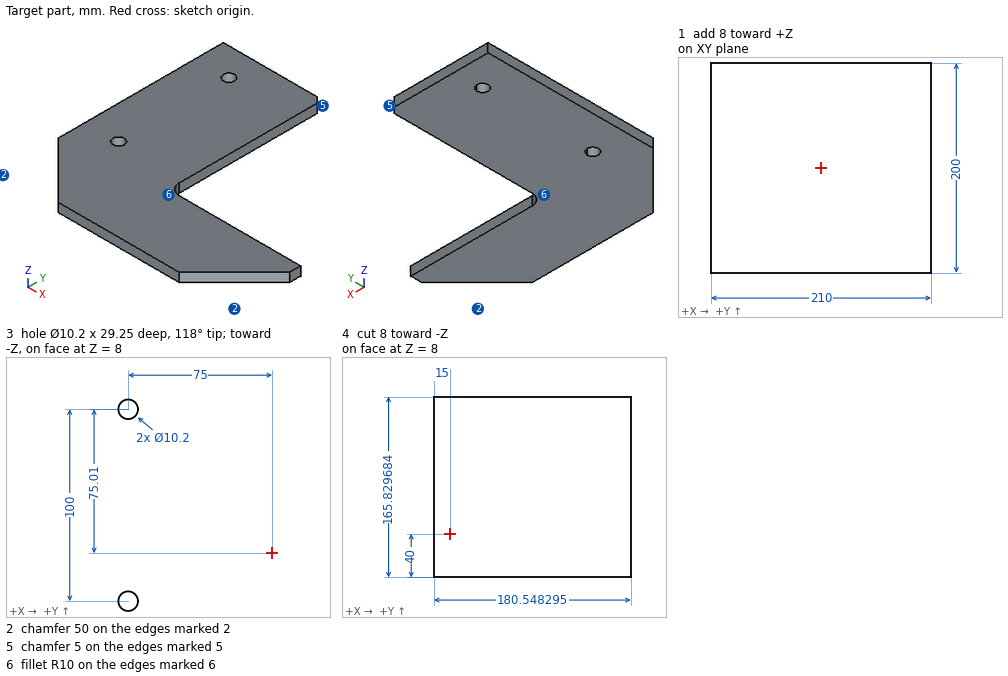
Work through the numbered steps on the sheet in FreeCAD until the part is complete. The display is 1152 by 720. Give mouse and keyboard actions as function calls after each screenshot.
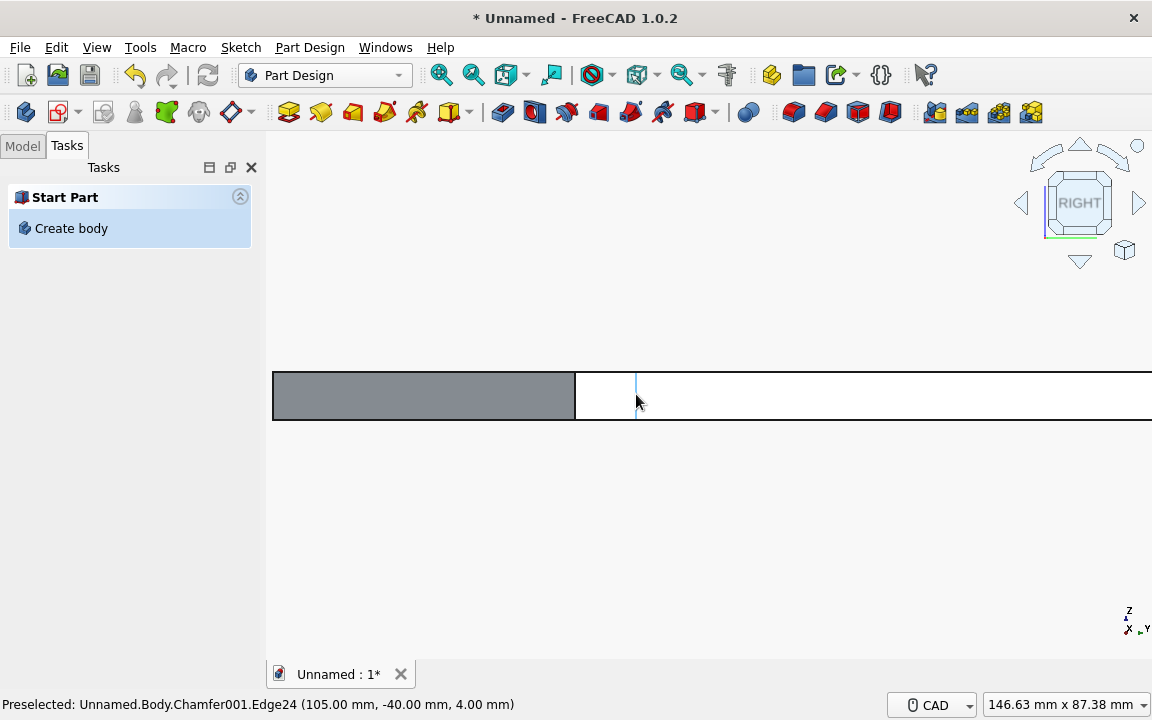
click(442, 76)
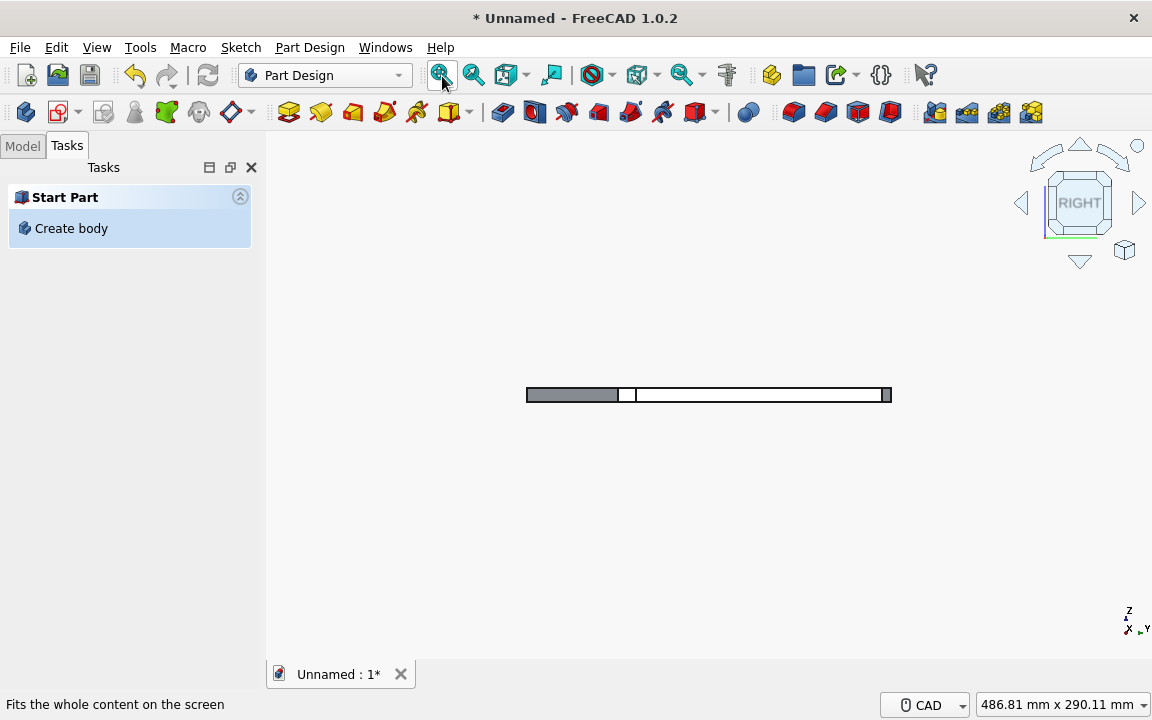
key(5)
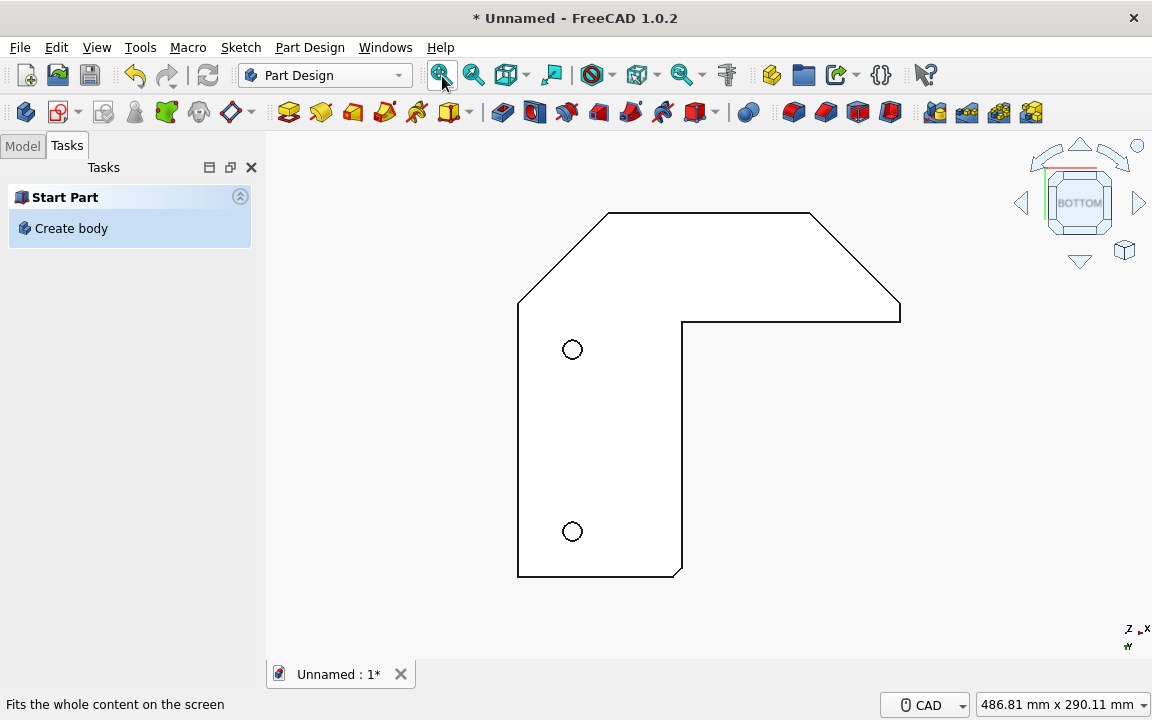
scroll(682, 321, up, 6)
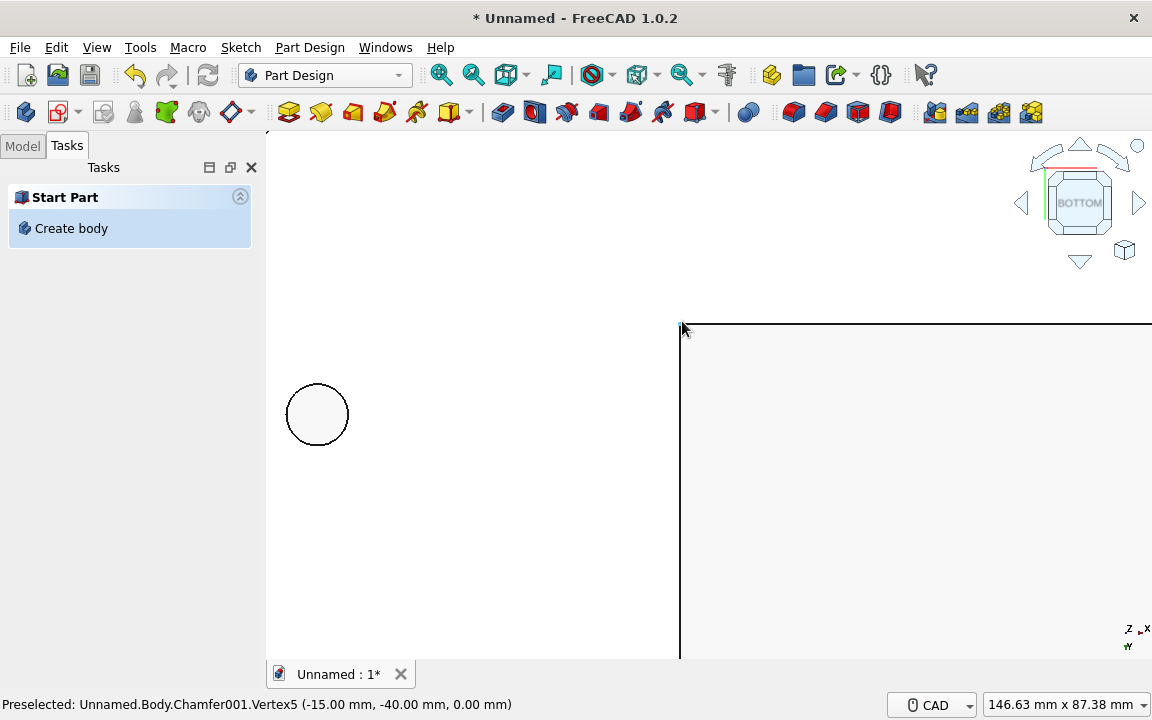
click(442, 76)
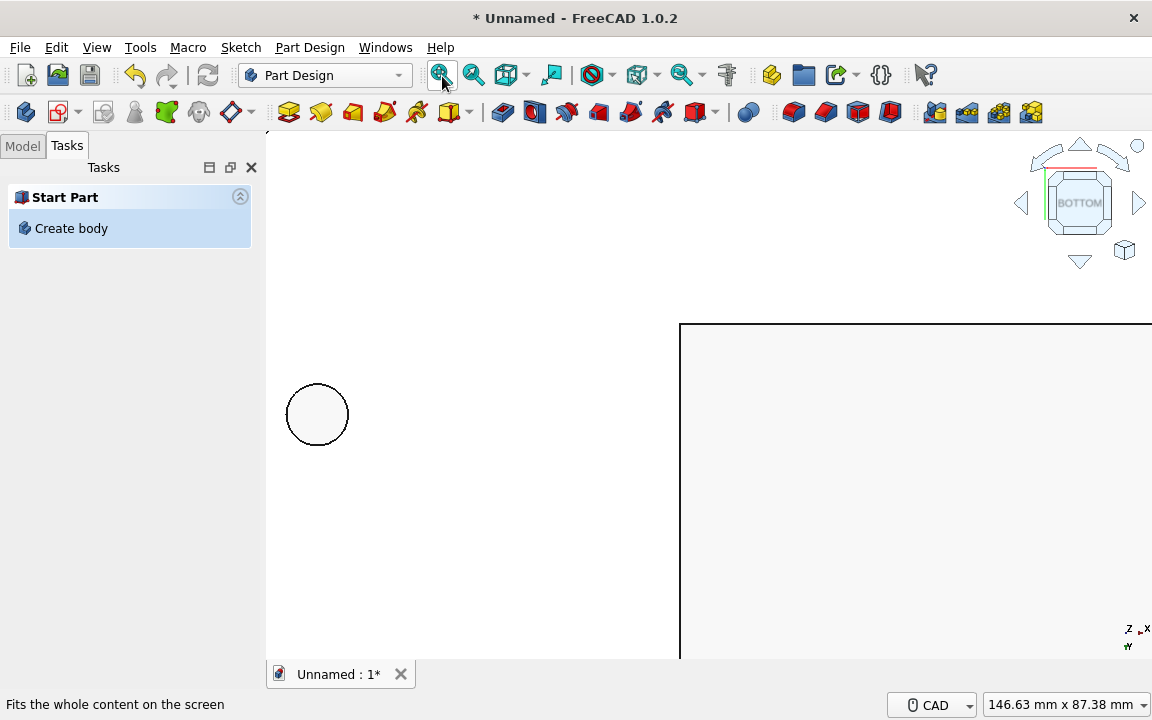
key(4)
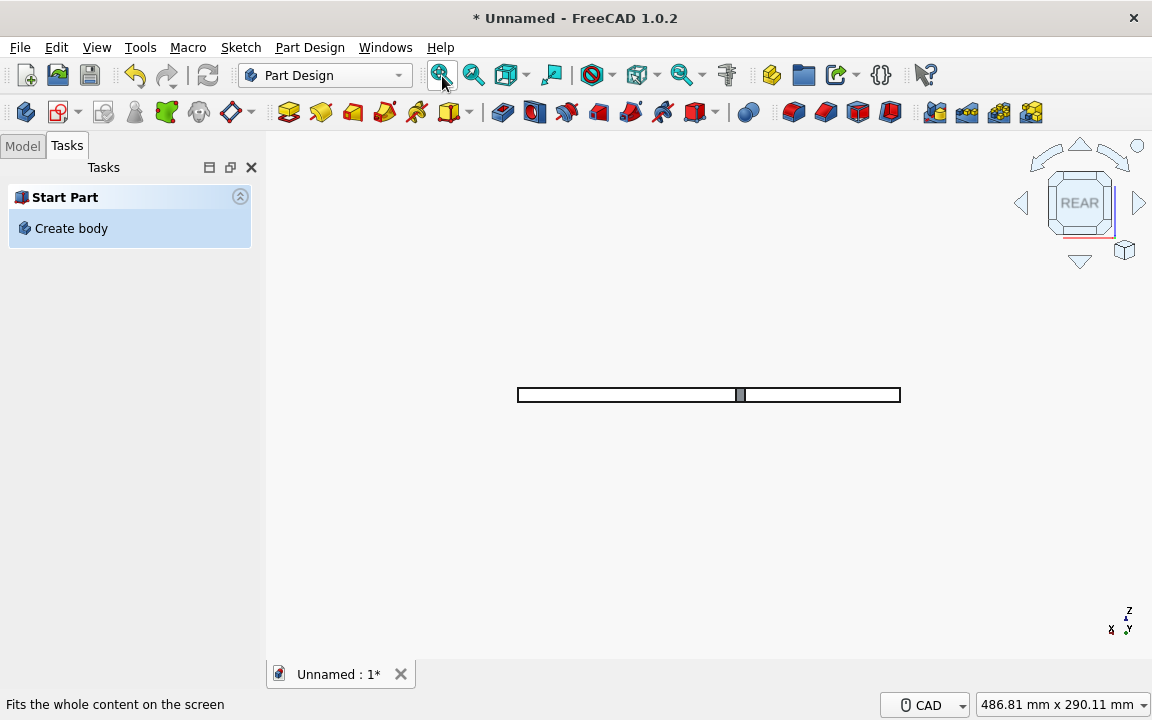
key(v)
key(f)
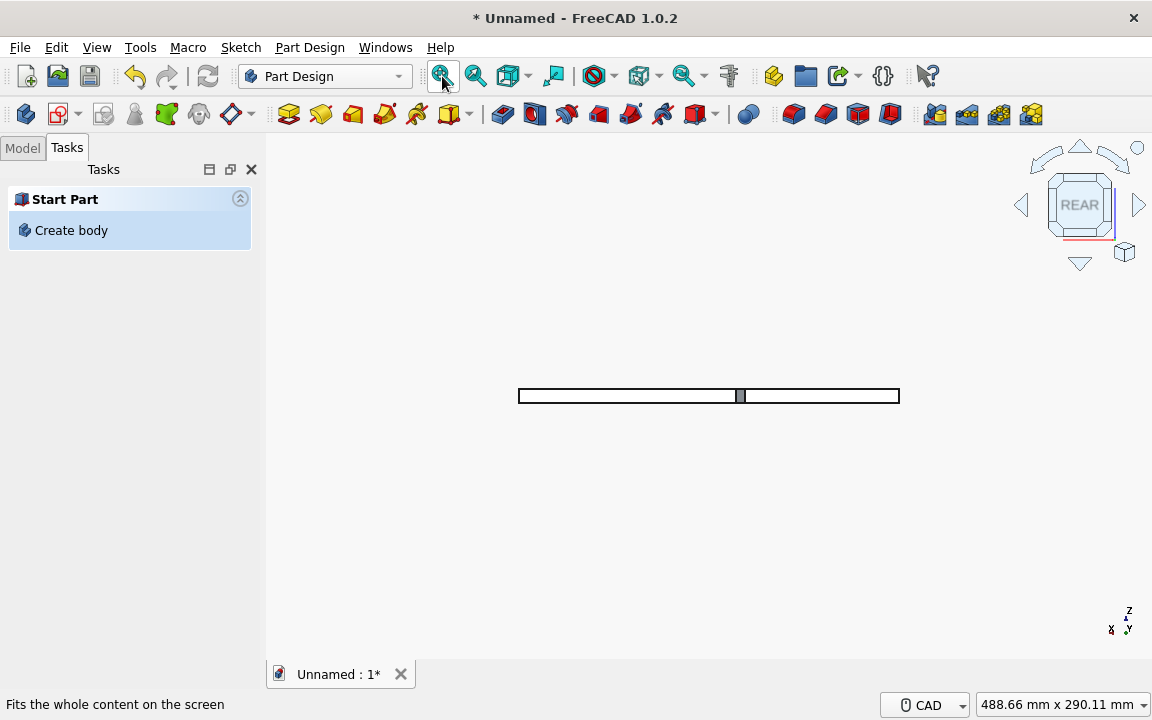
scroll(736, 395, up, 6)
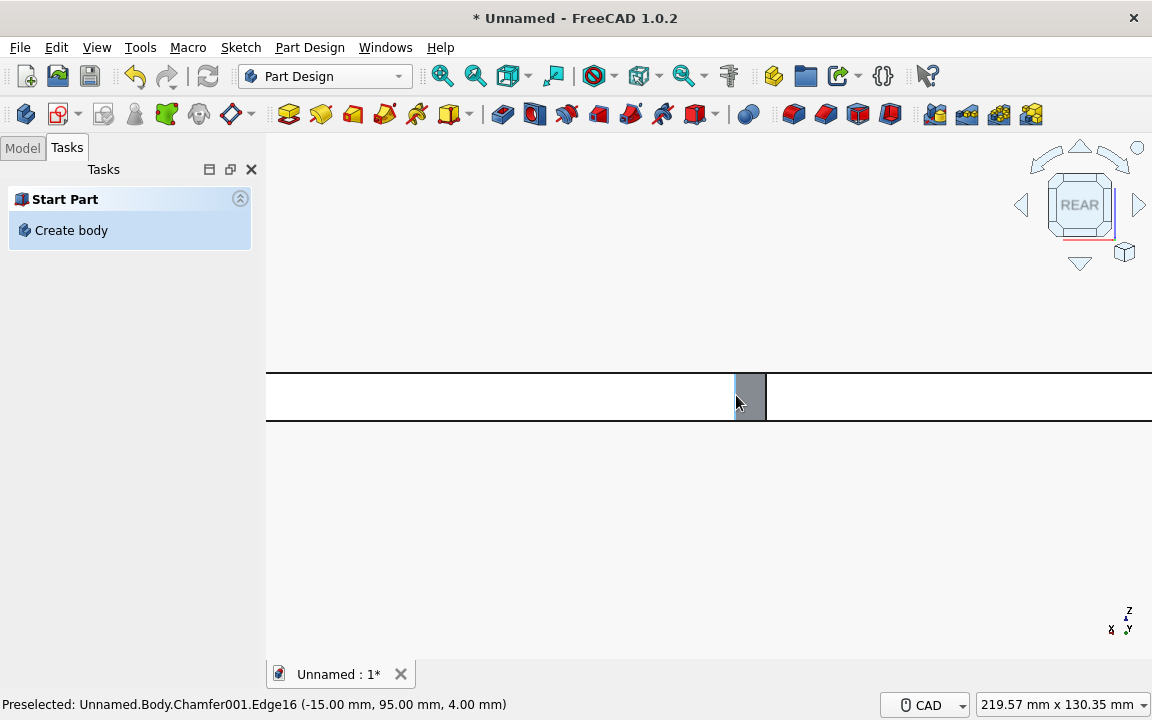
key(v)
key(f)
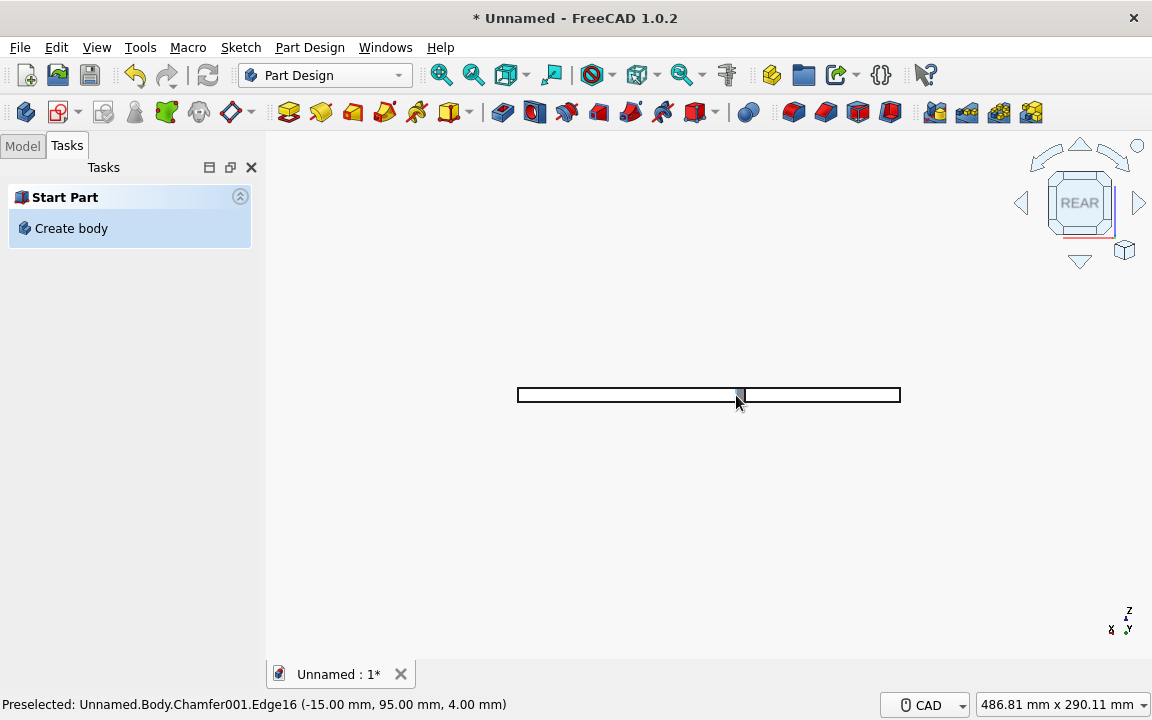
key(6)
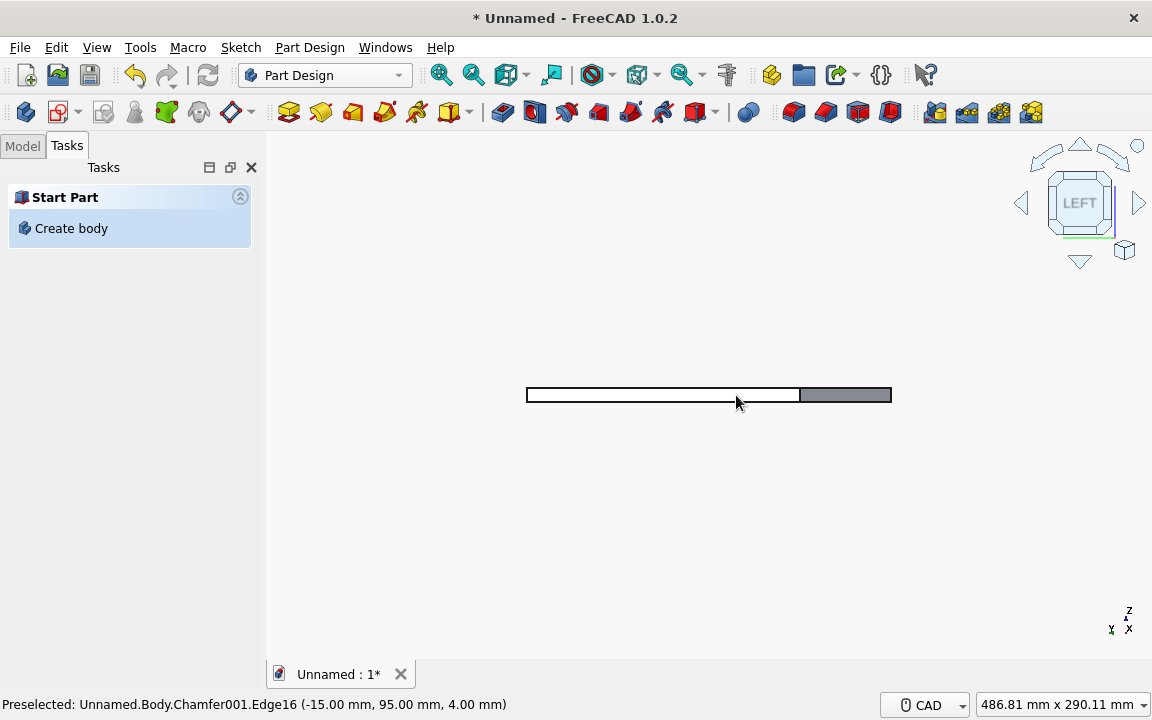
click(442, 76)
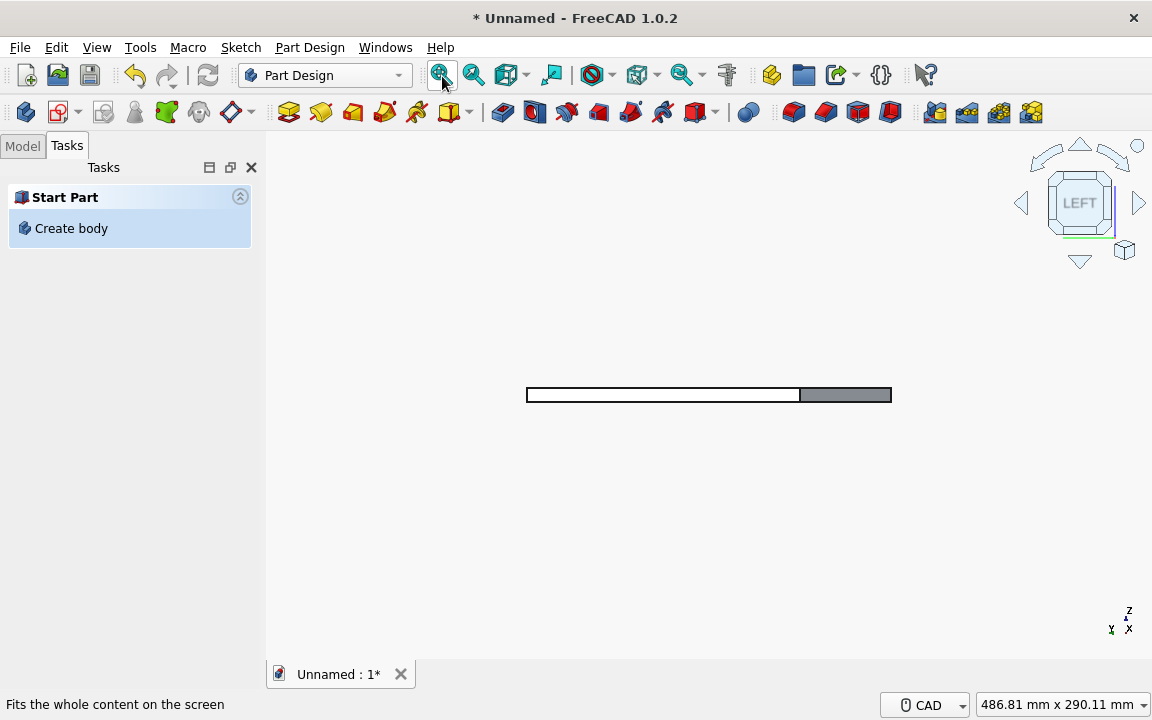
scroll(782, 394, up, 6)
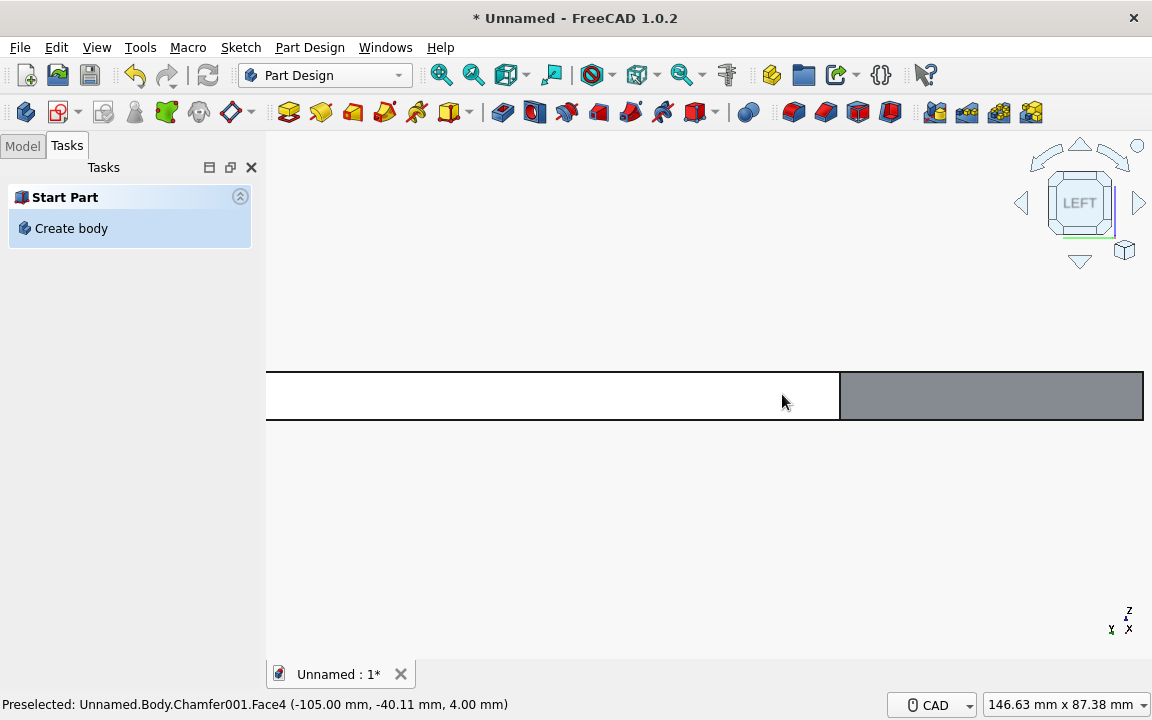
key(v)
key(f)